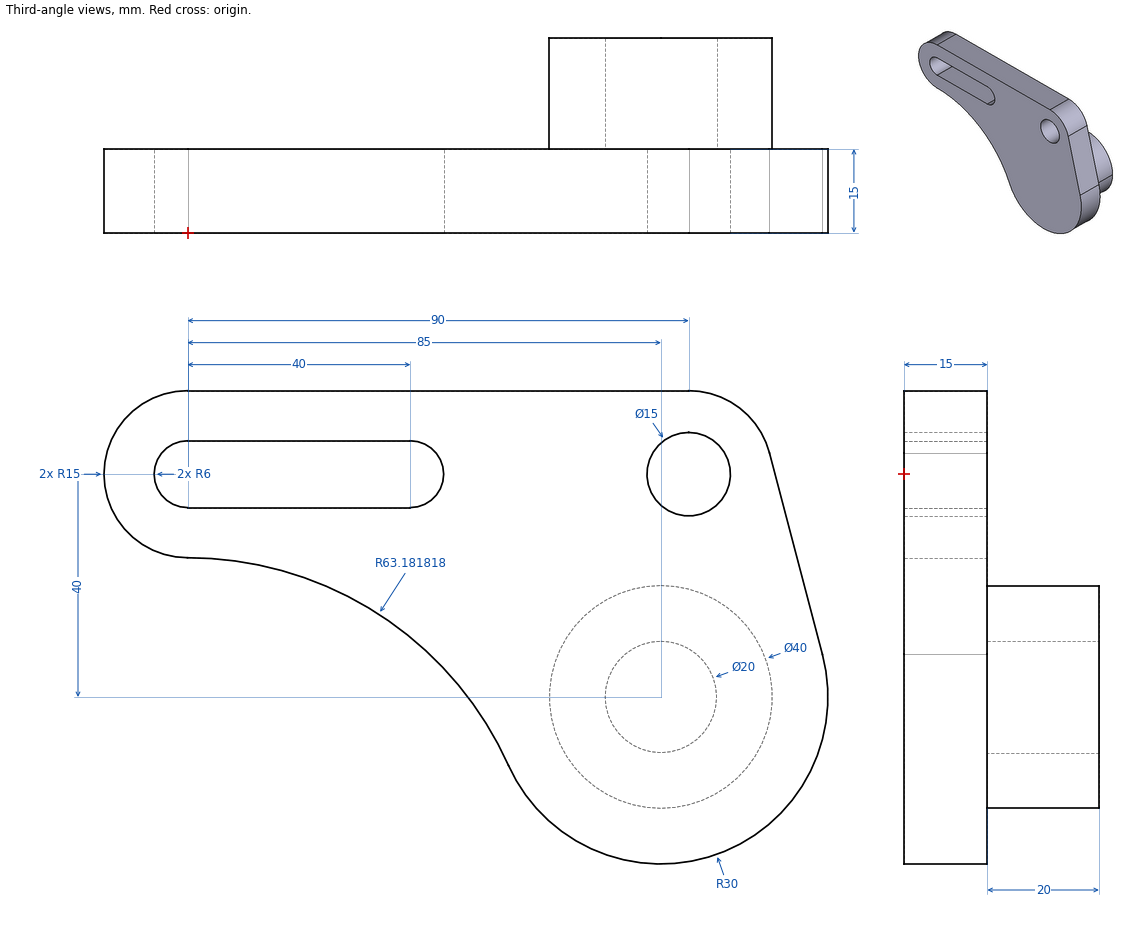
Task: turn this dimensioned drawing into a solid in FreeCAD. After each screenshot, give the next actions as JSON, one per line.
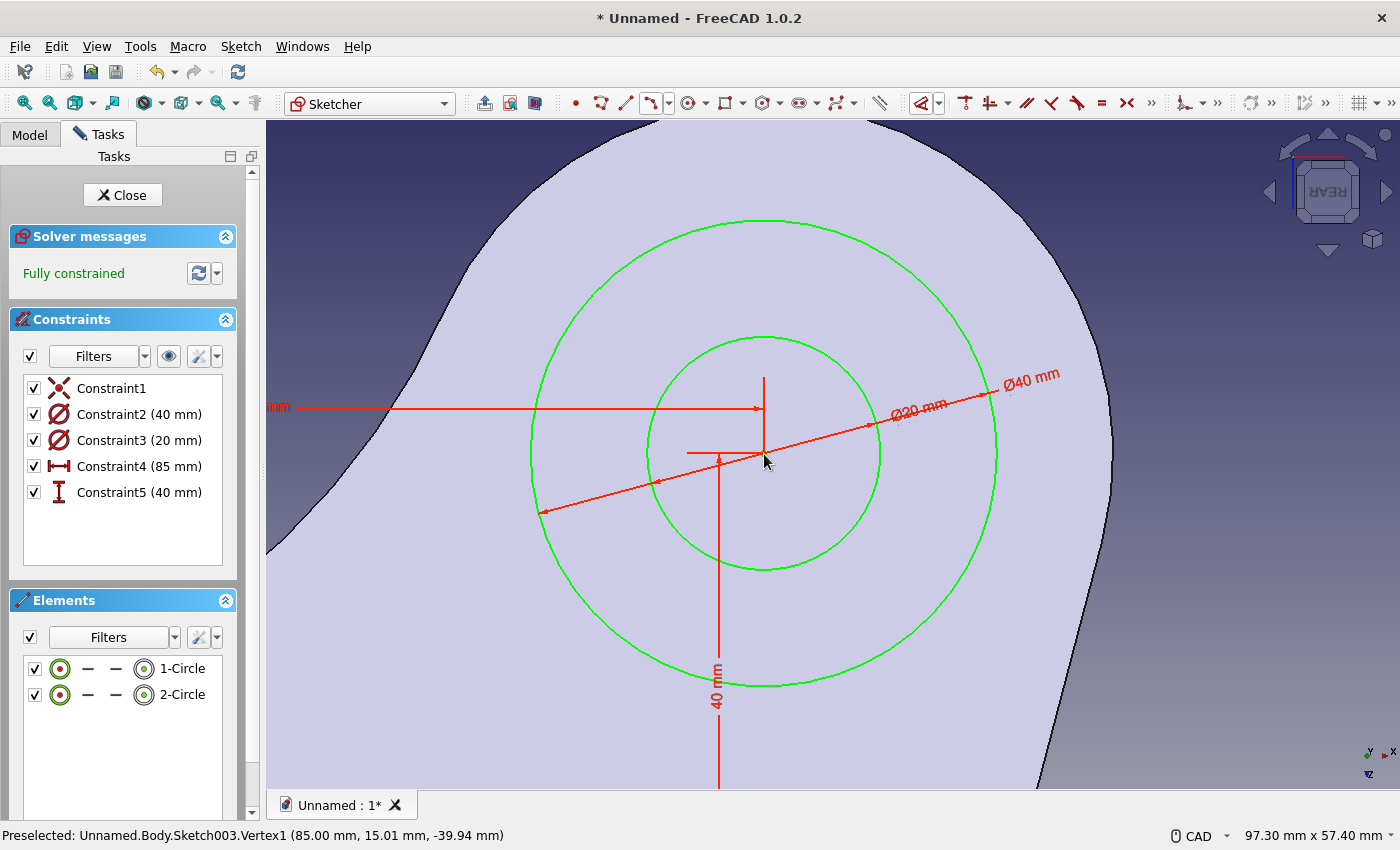
{"action": "left_click", "coordinate": [123, 195]}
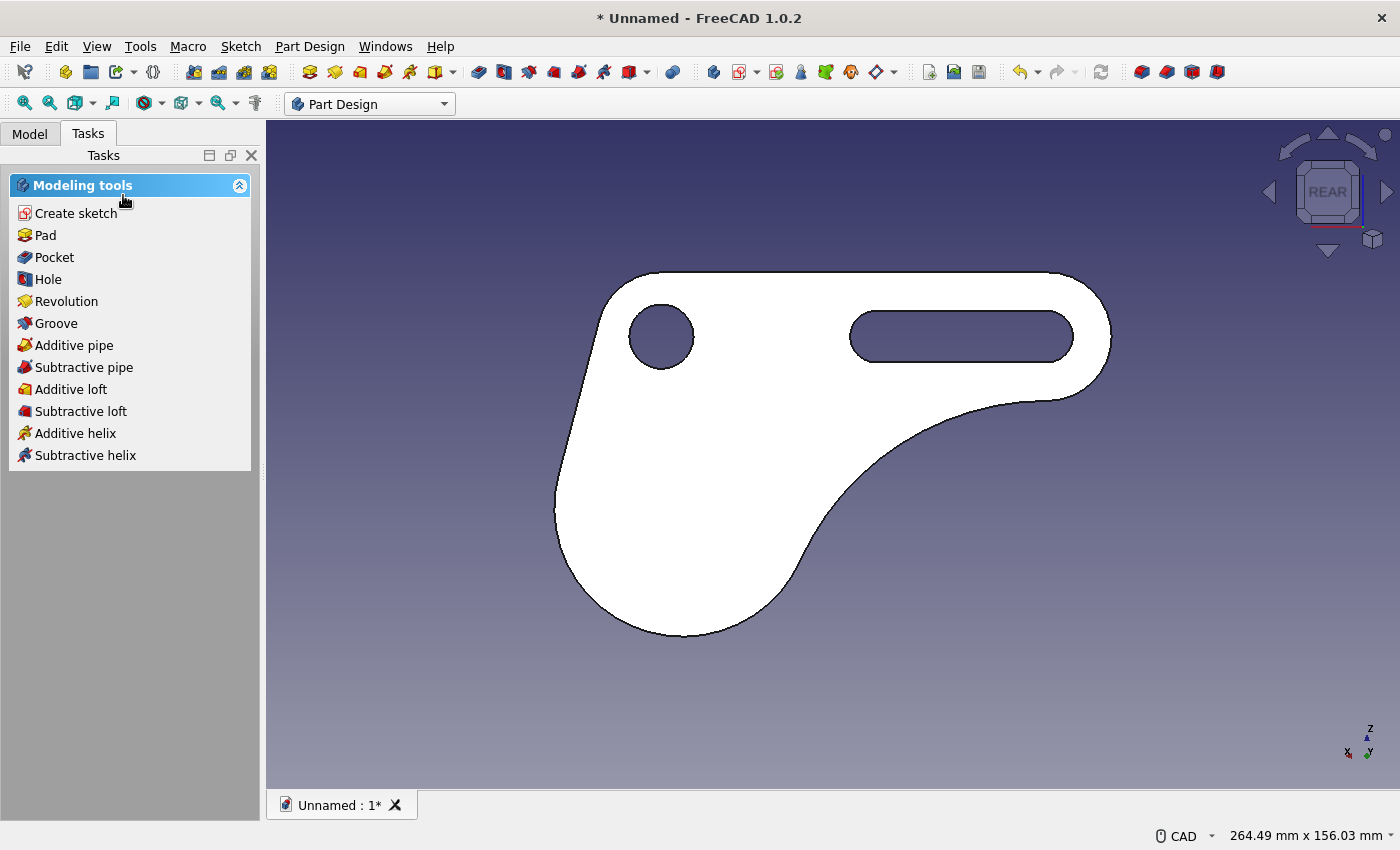
{"action": "left_click", "coordinate": [310, 72]}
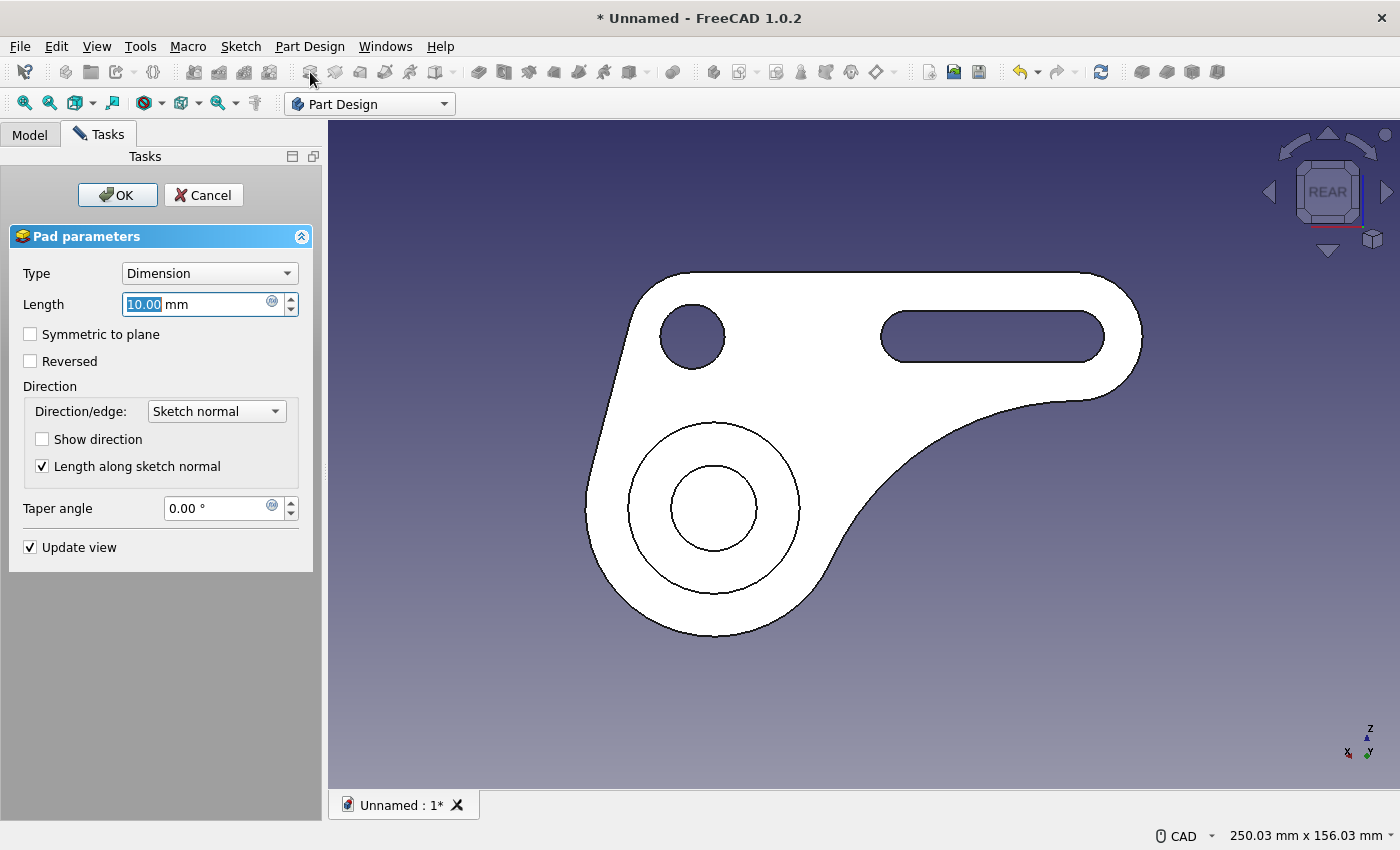
{"action": "type", "text": "20"}
{"action": "key", "text": "Tab"}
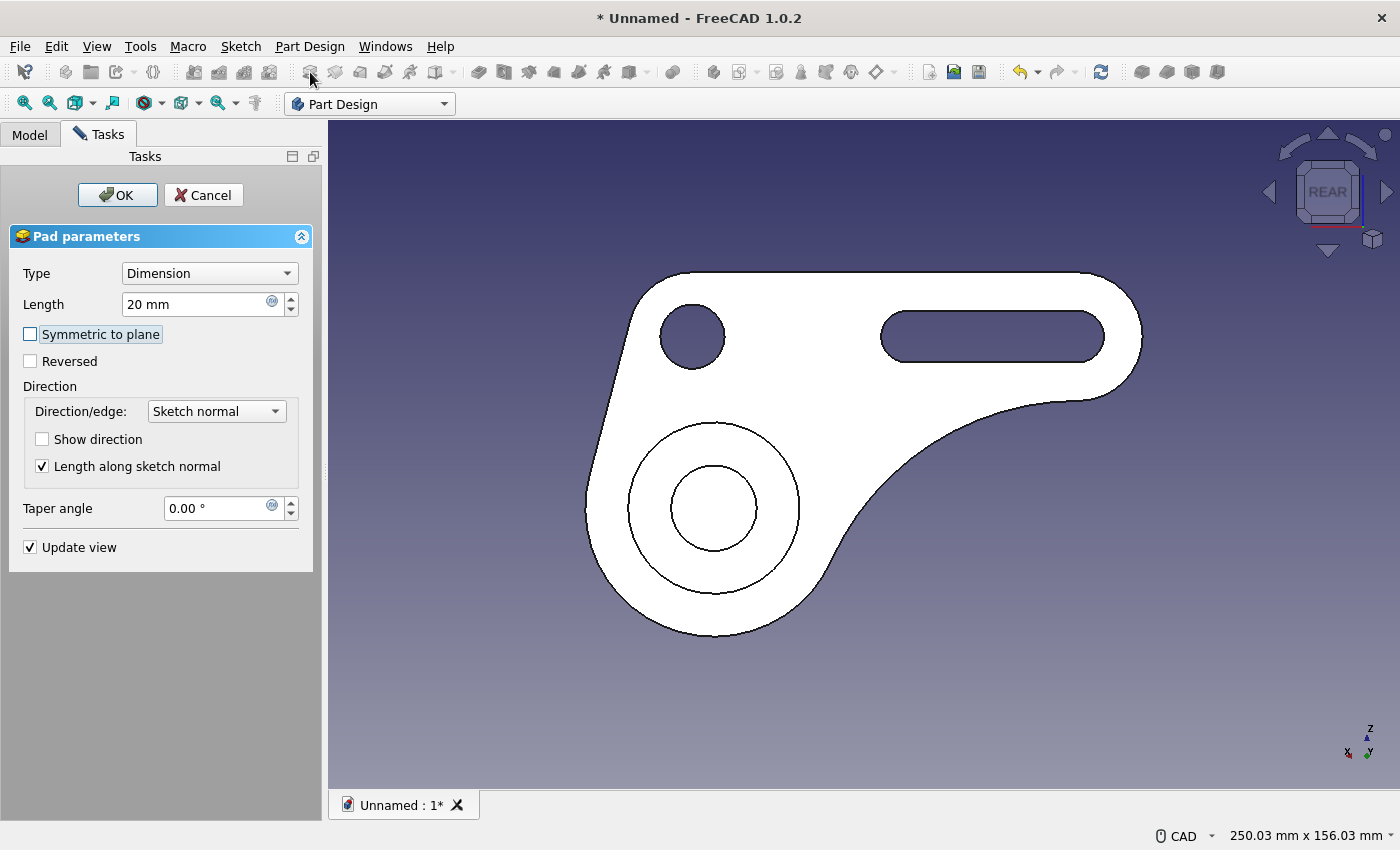
{"action": "left_click", "coordinate": [118, 195]}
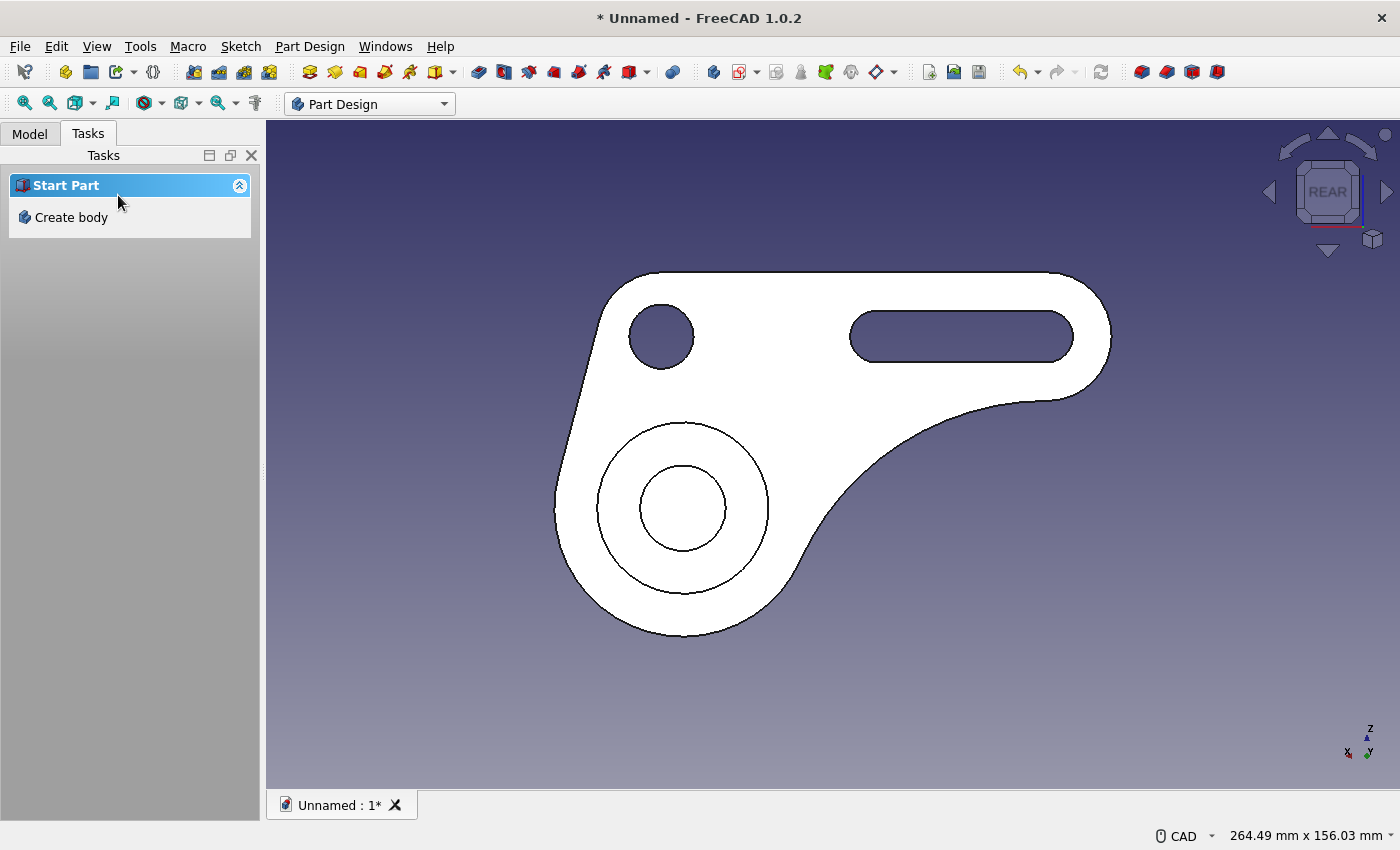
{"action": "key", "text": "0"}